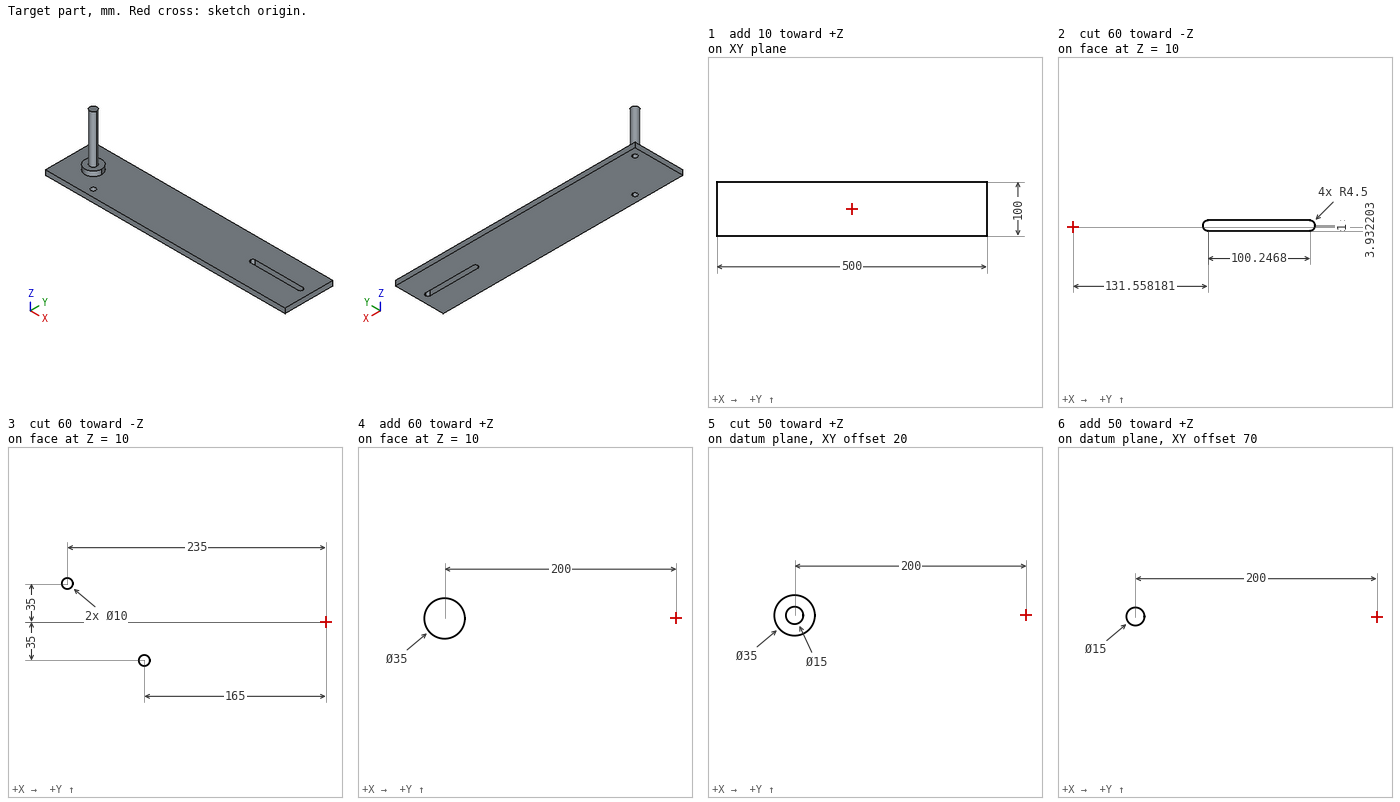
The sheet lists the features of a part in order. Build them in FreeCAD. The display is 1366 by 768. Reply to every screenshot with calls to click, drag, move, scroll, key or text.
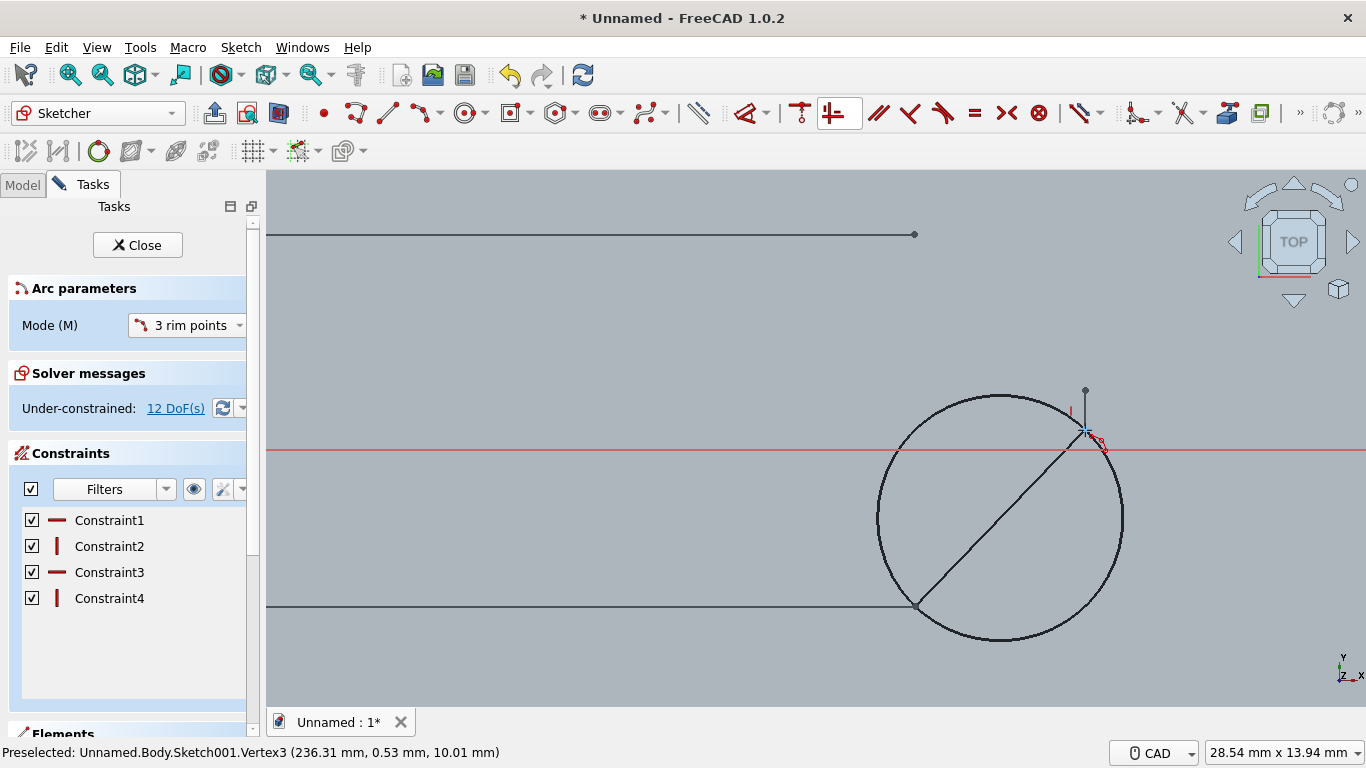
scroll(1086, 441, down, 13)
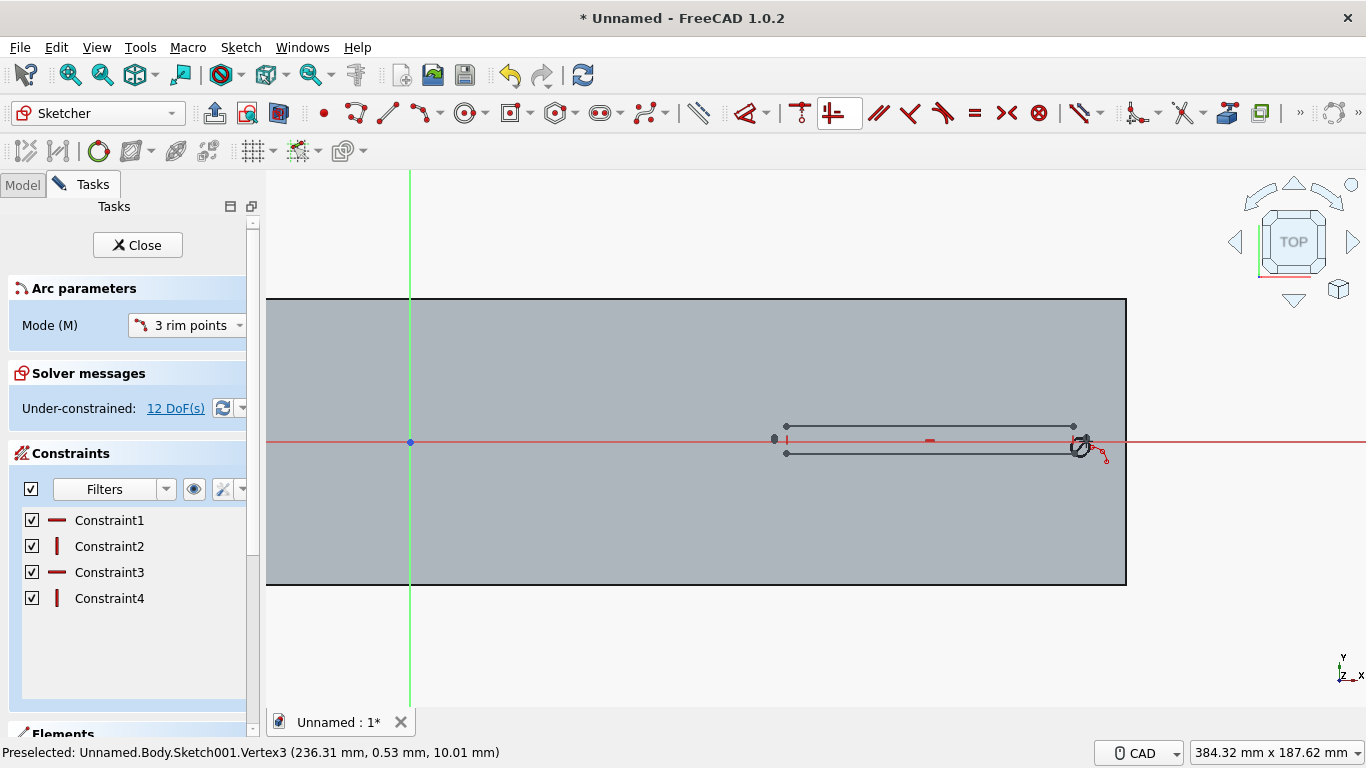
scroll(1083, 450, up, 8)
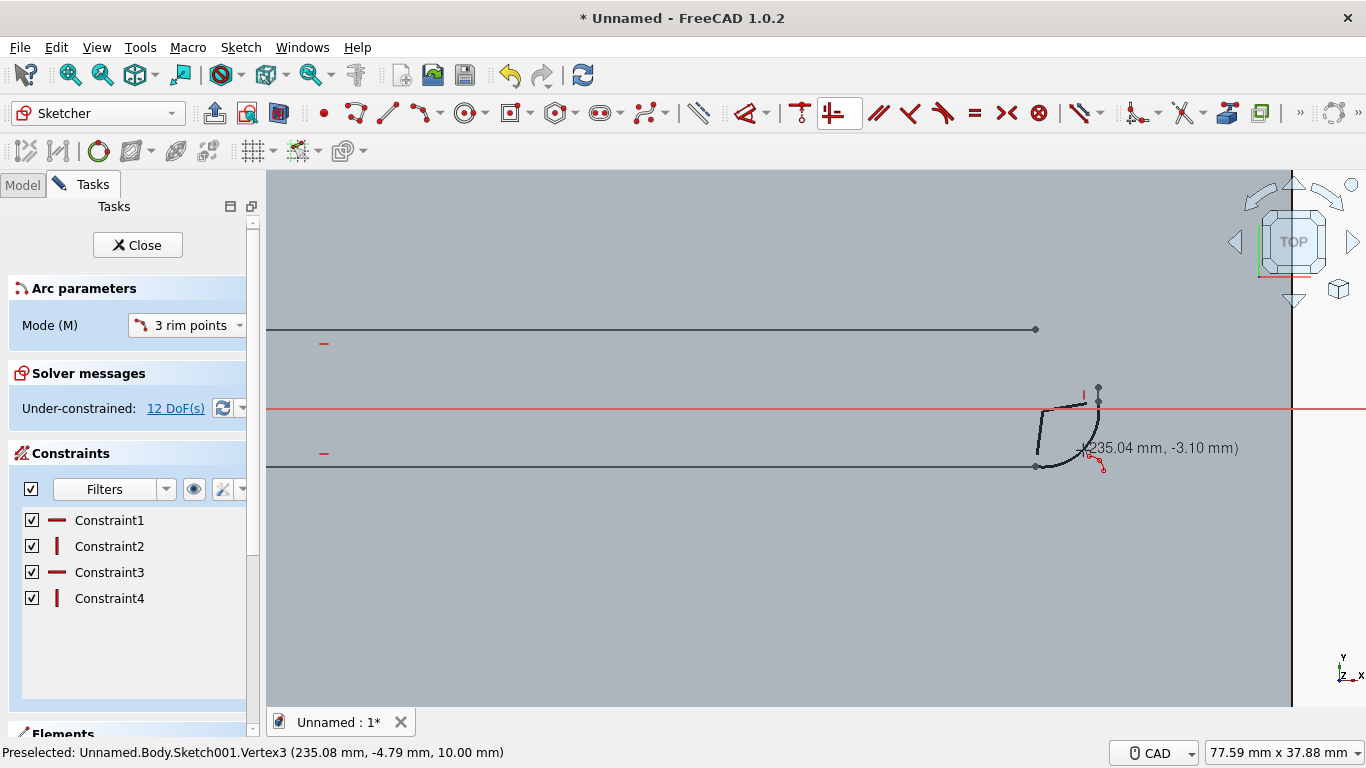
click(1079, 446)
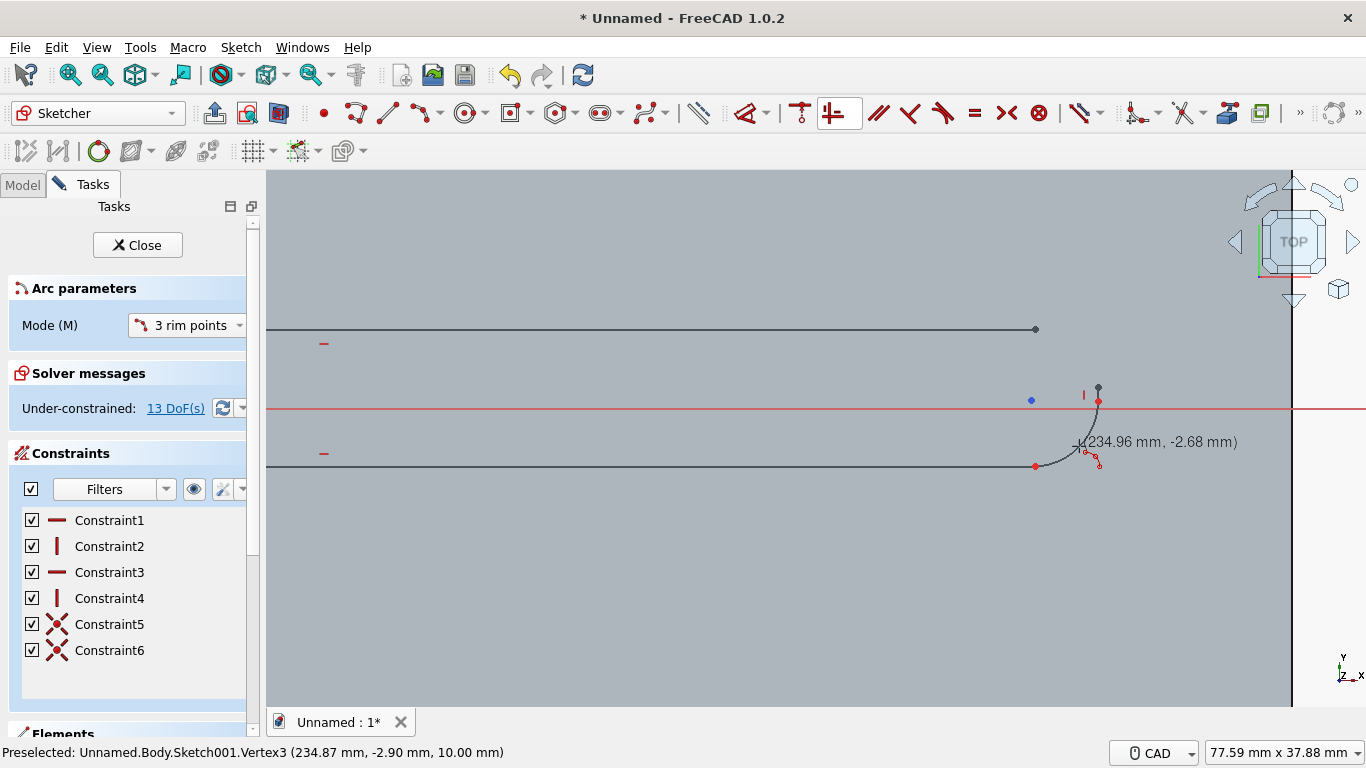
scroll(1098, 387, up, 5)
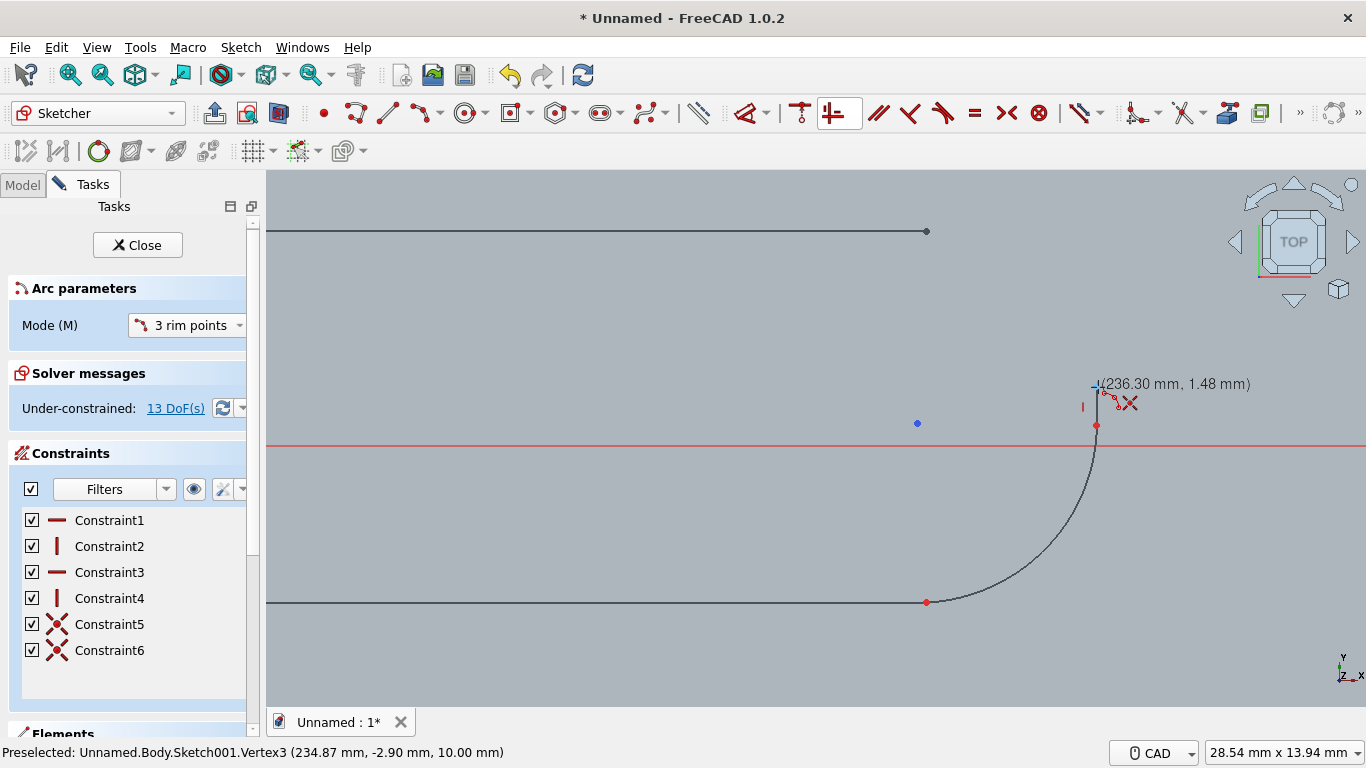
click(1097, 387)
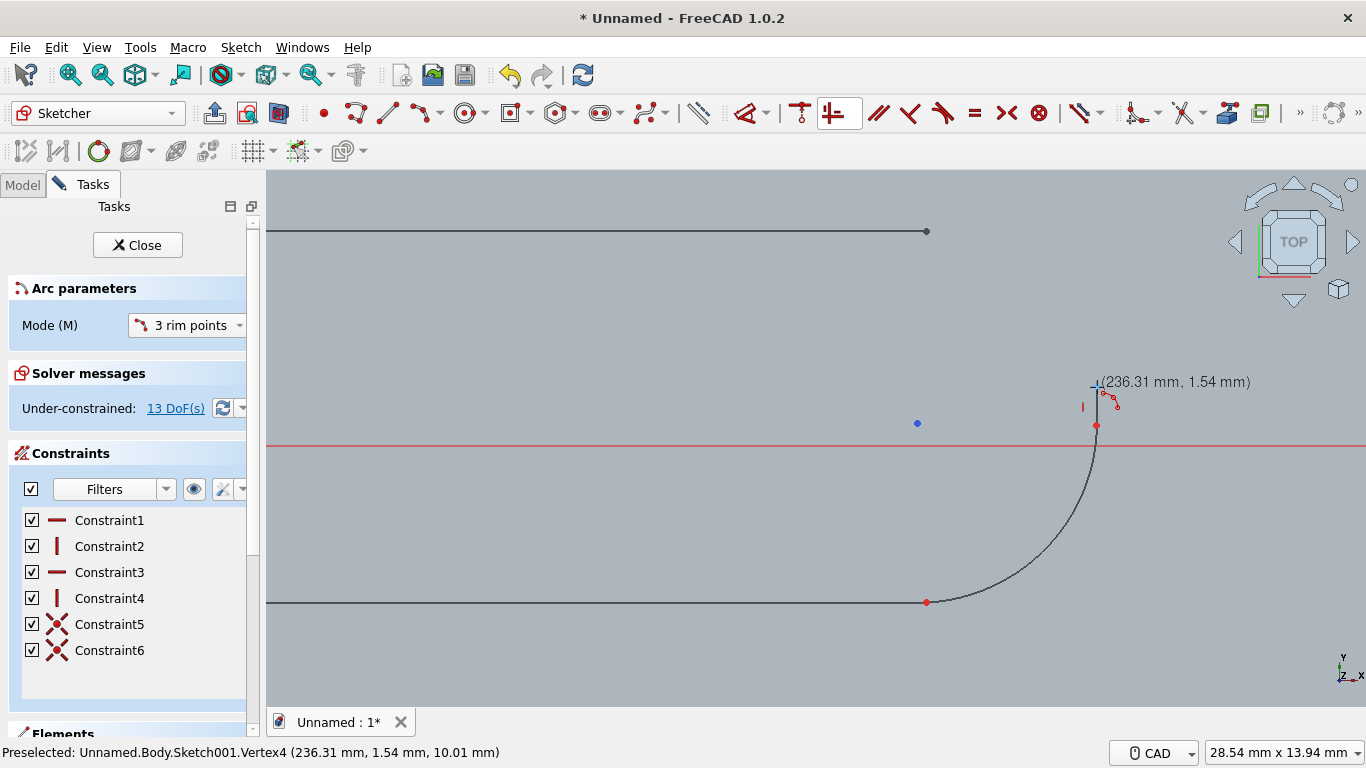
scroll(1085, 441, down, 13)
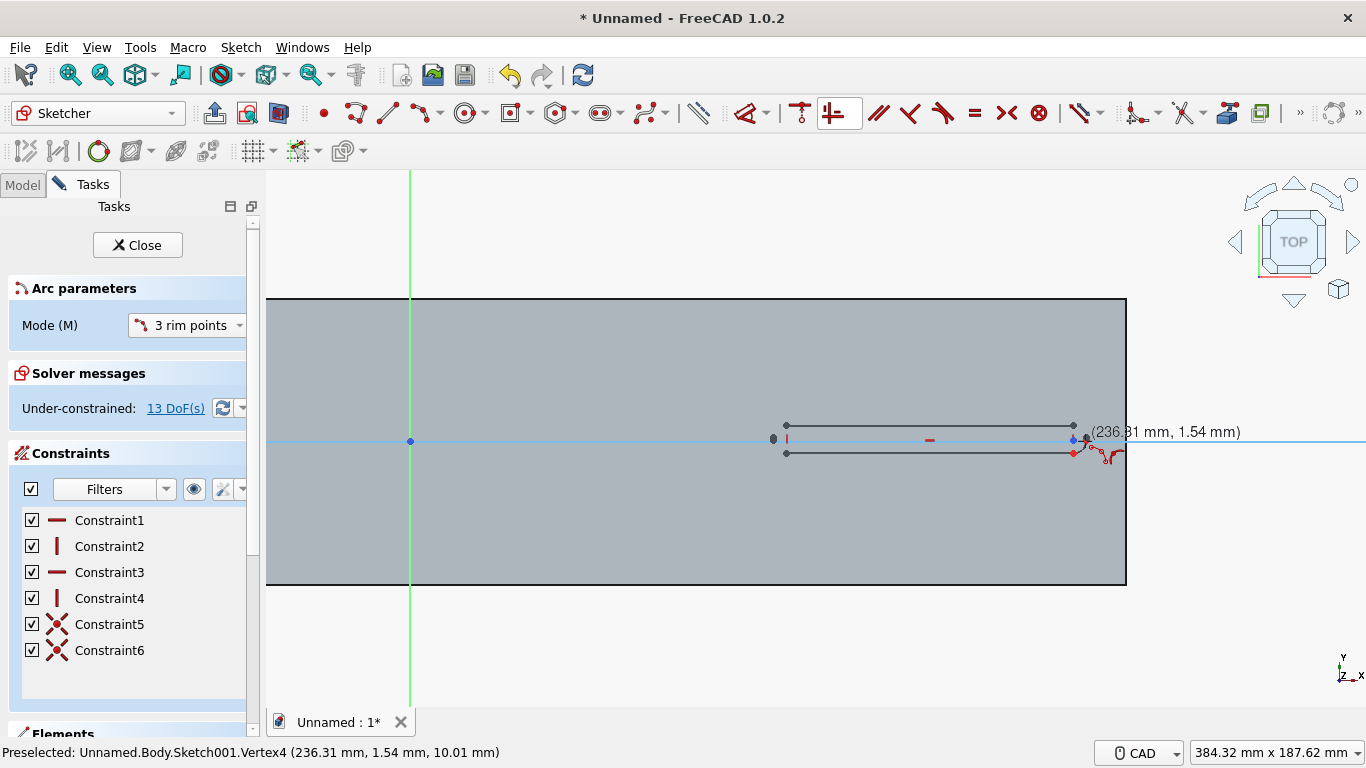
click(1074, 426)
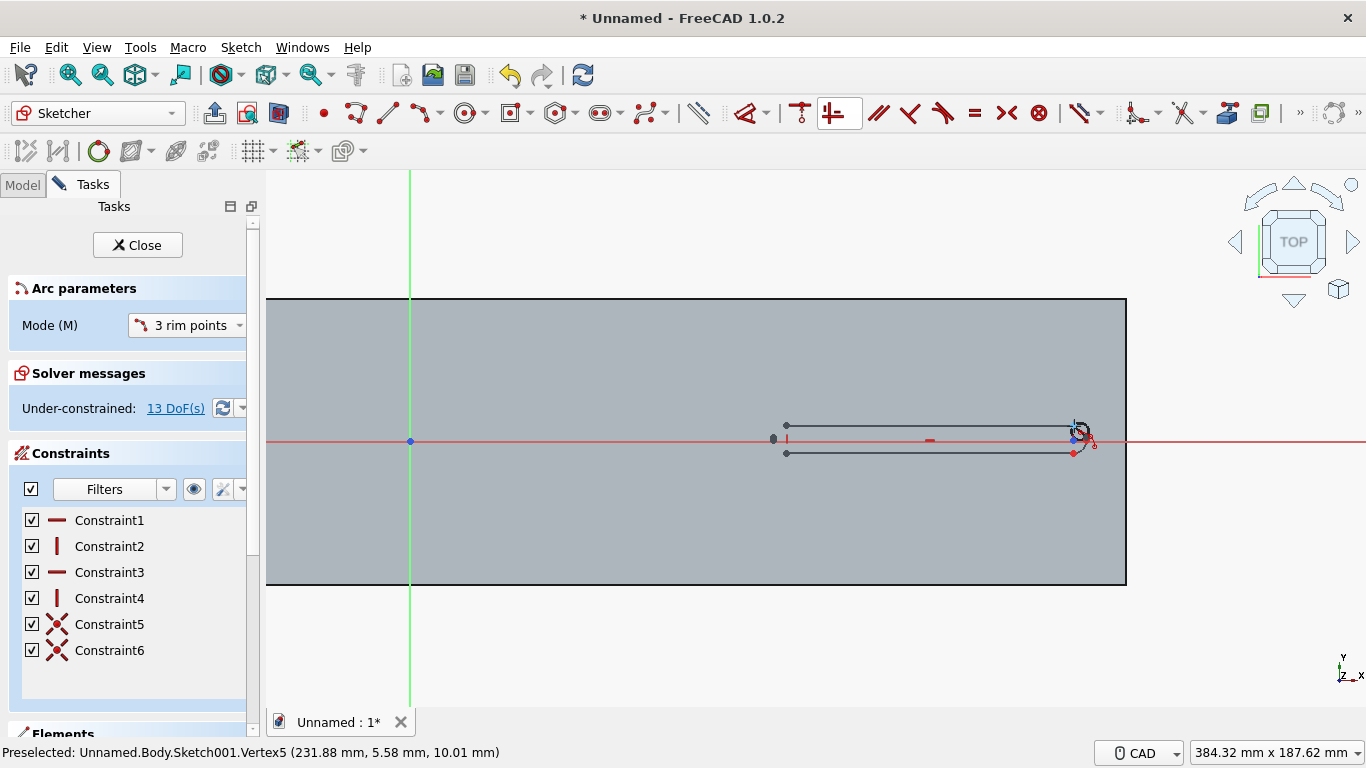
scroll(1083, 428, up, 8)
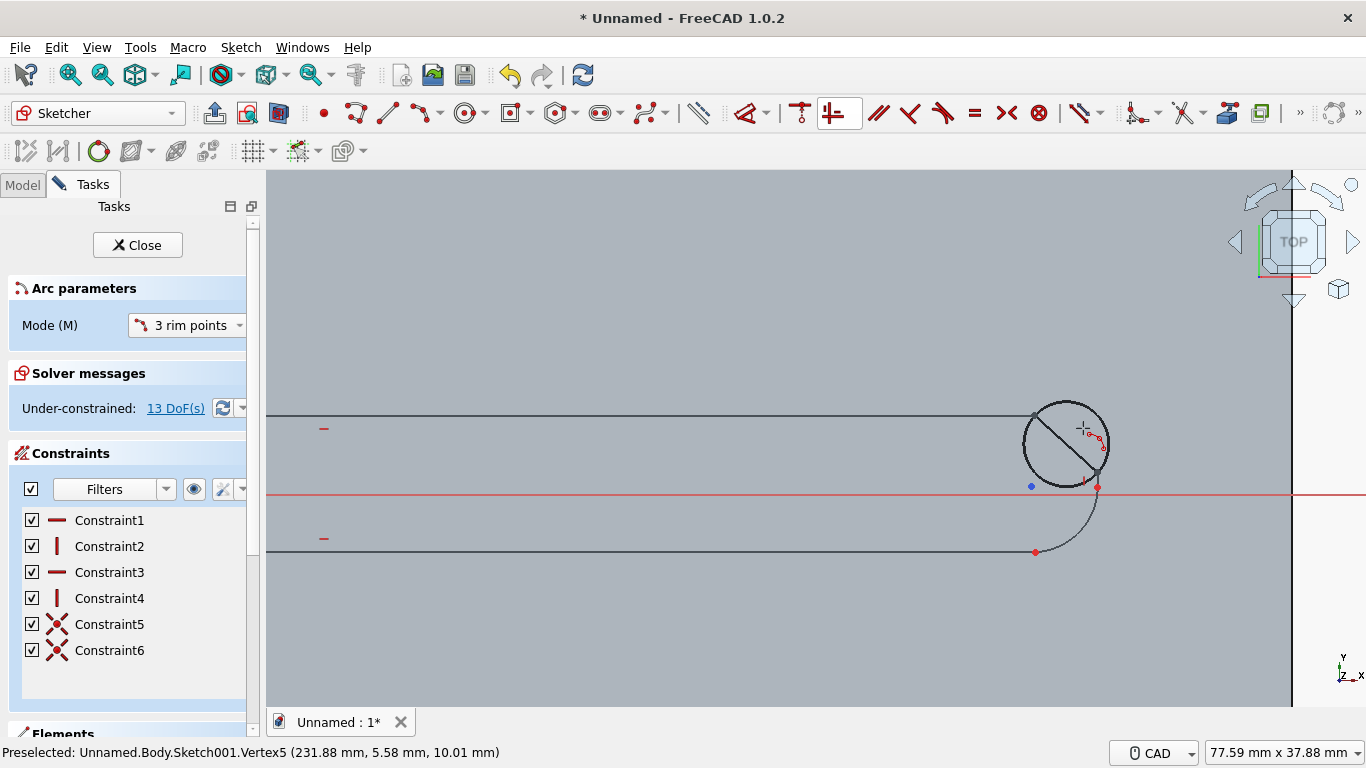
click(1079, 427)